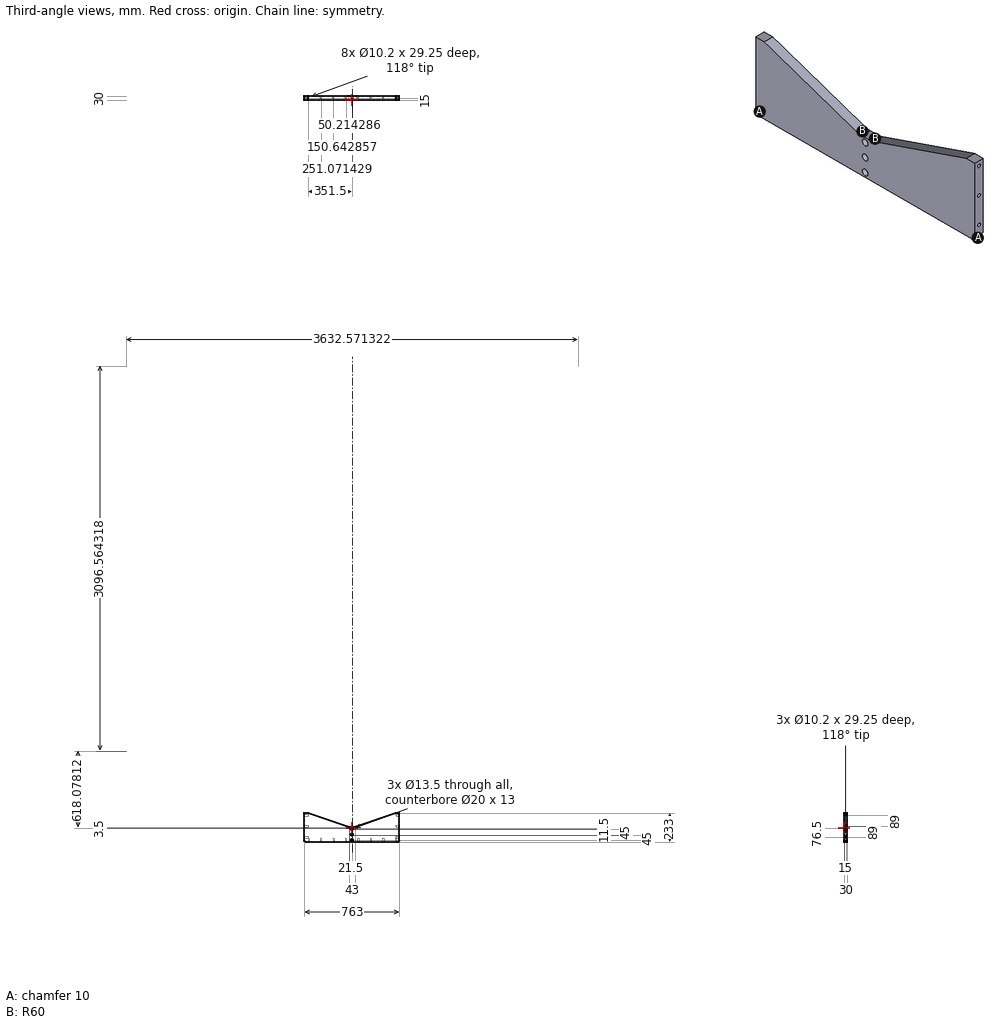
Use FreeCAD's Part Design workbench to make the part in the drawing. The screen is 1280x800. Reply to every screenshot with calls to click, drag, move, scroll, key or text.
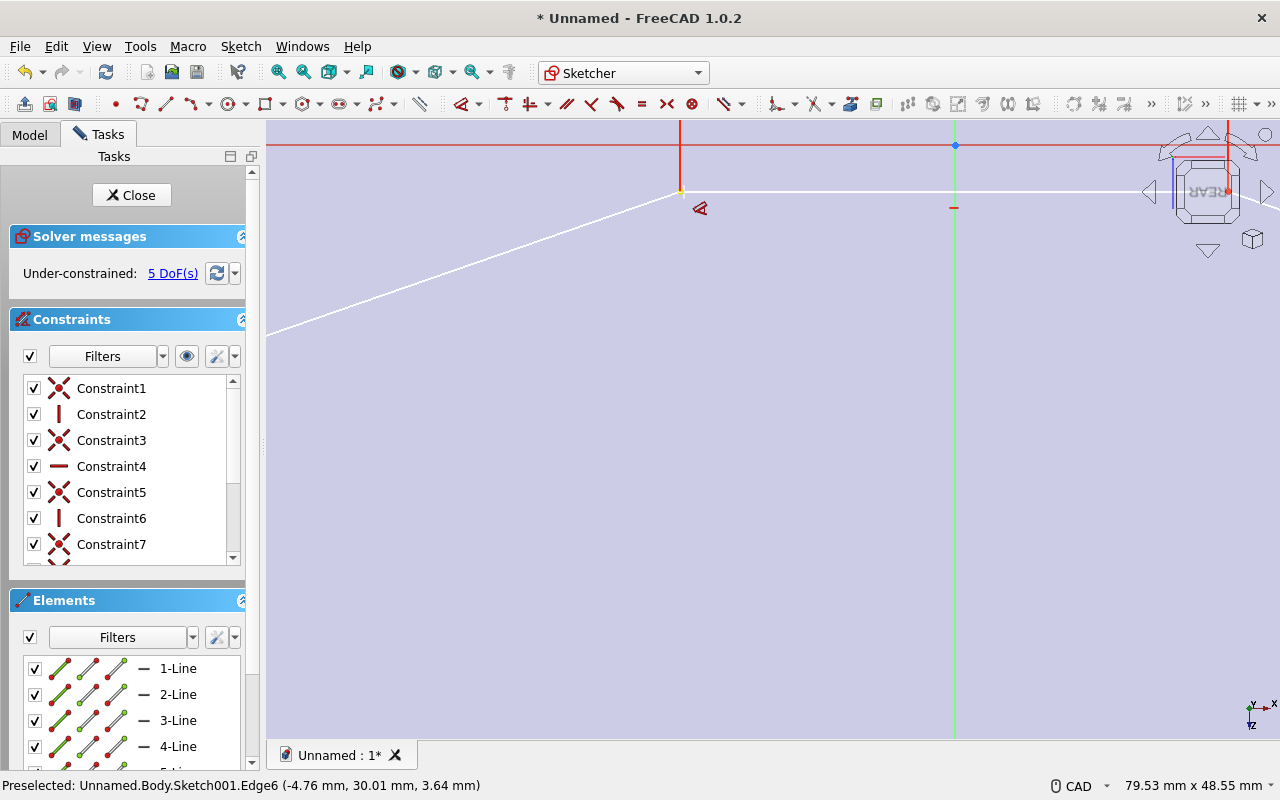
click(680, 192)
click(646, 170)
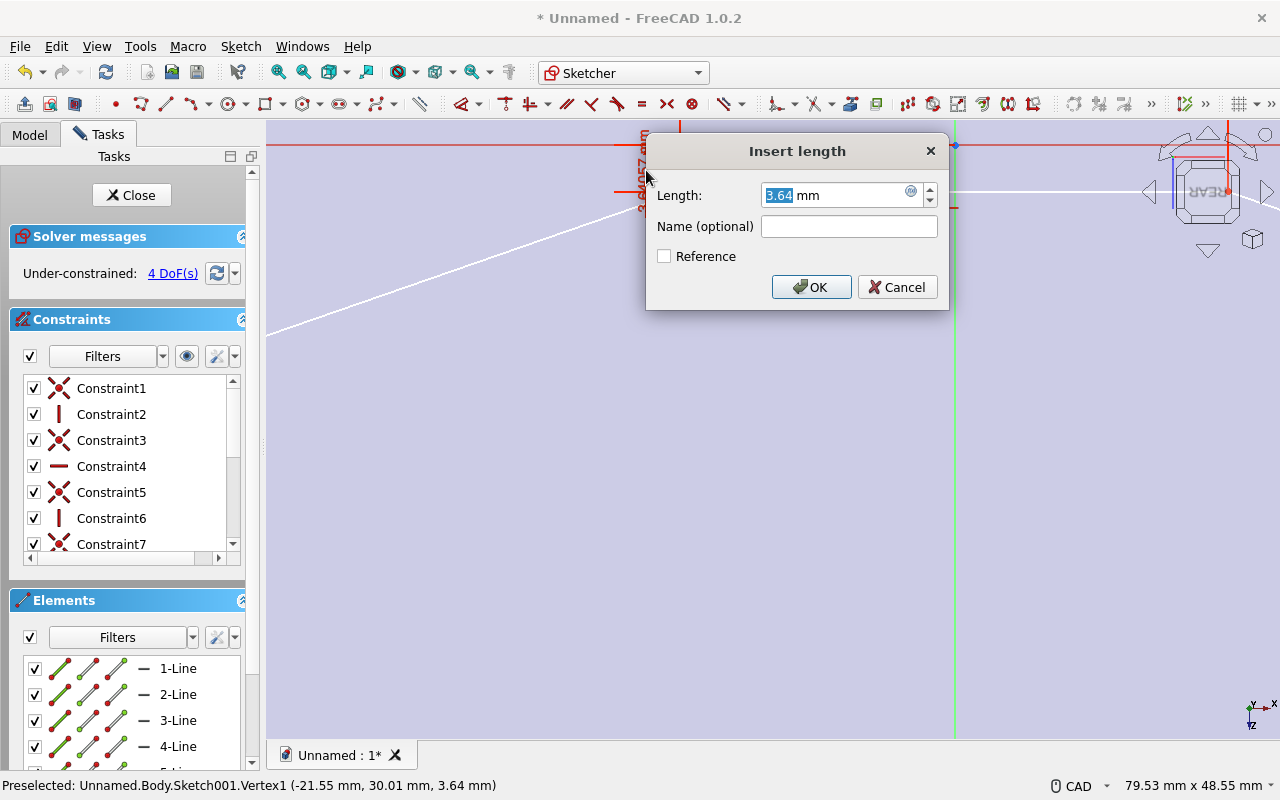
text(3.5)
key(Return)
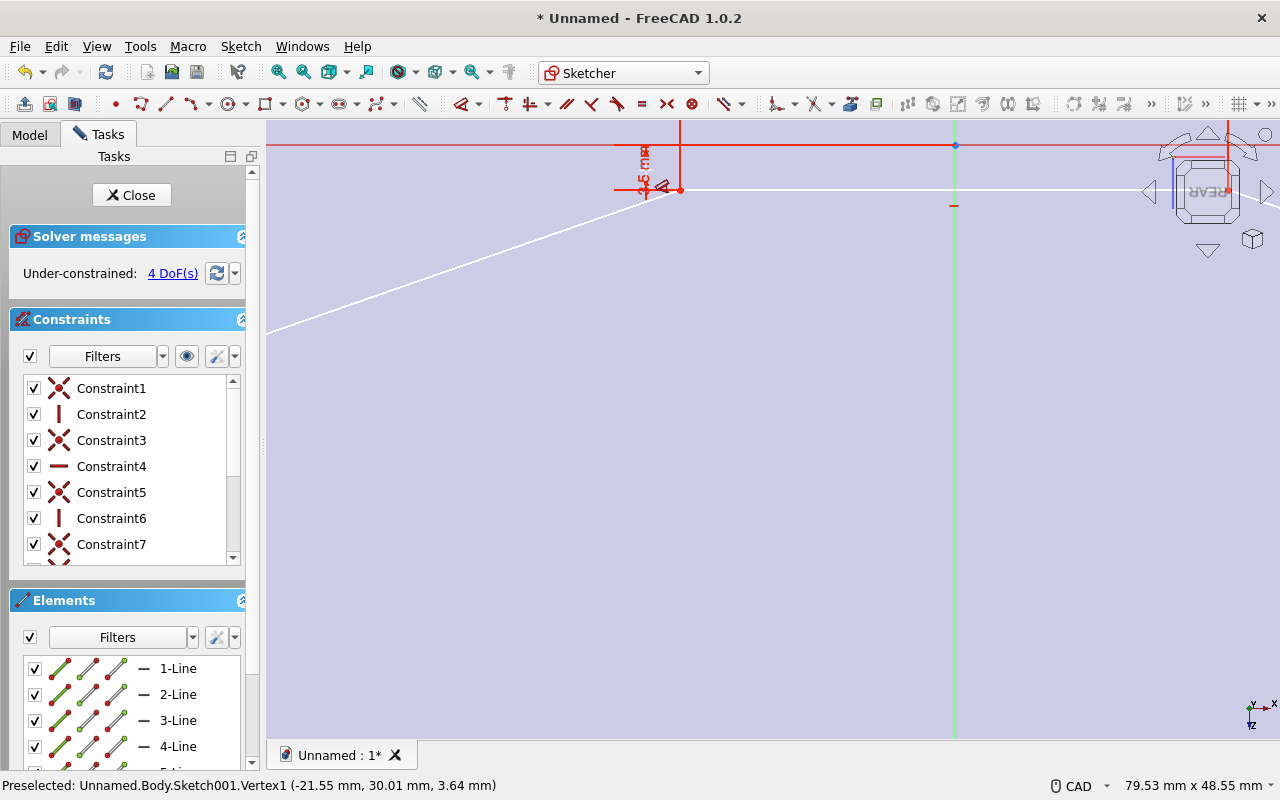
scroll(704, 430, down, 15)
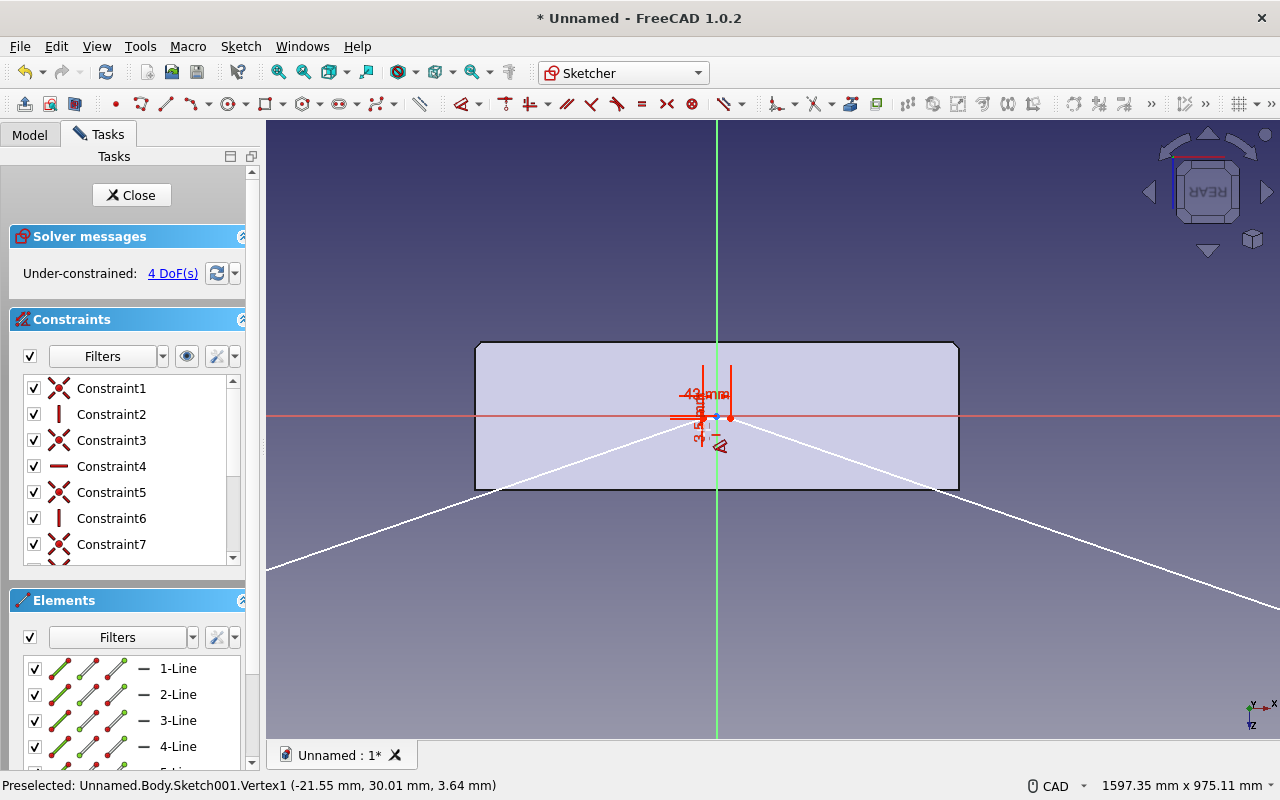
scroll(702, 199, down, 9)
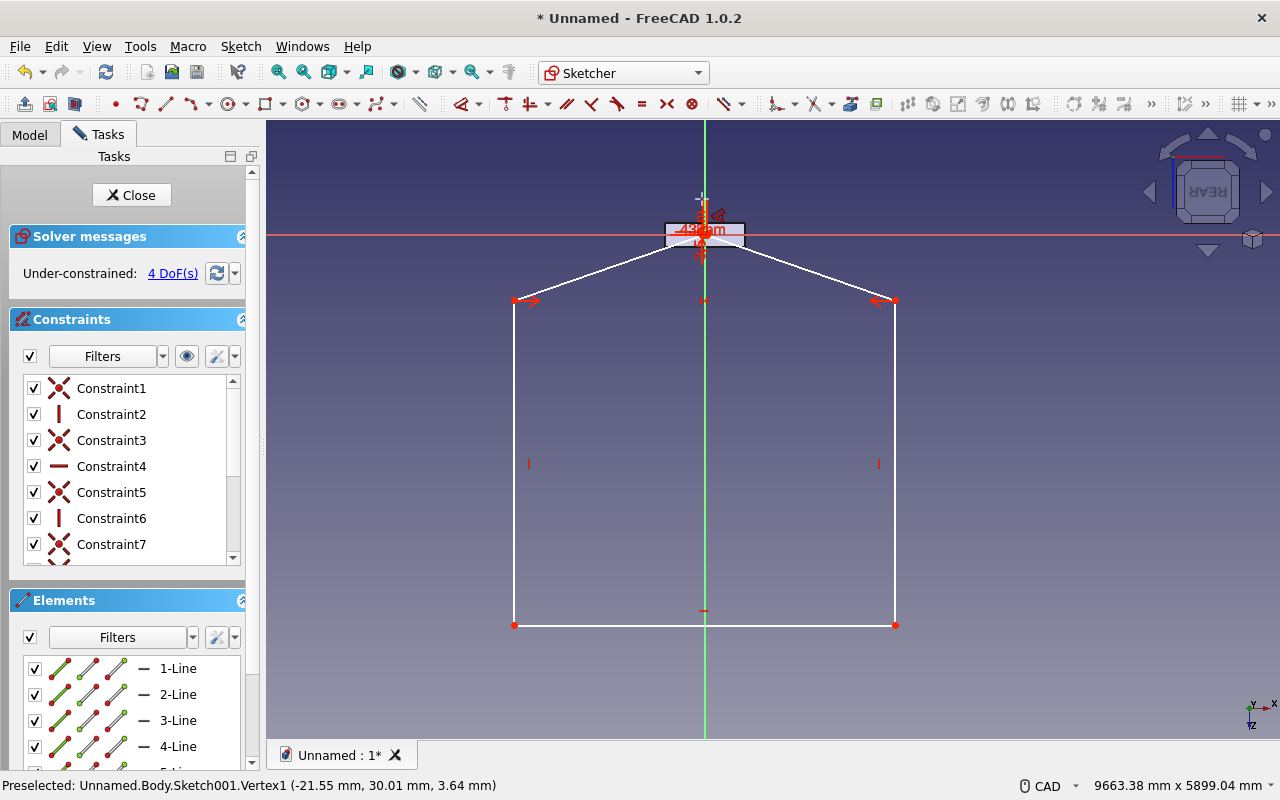
scroll(703, 235, up, 15)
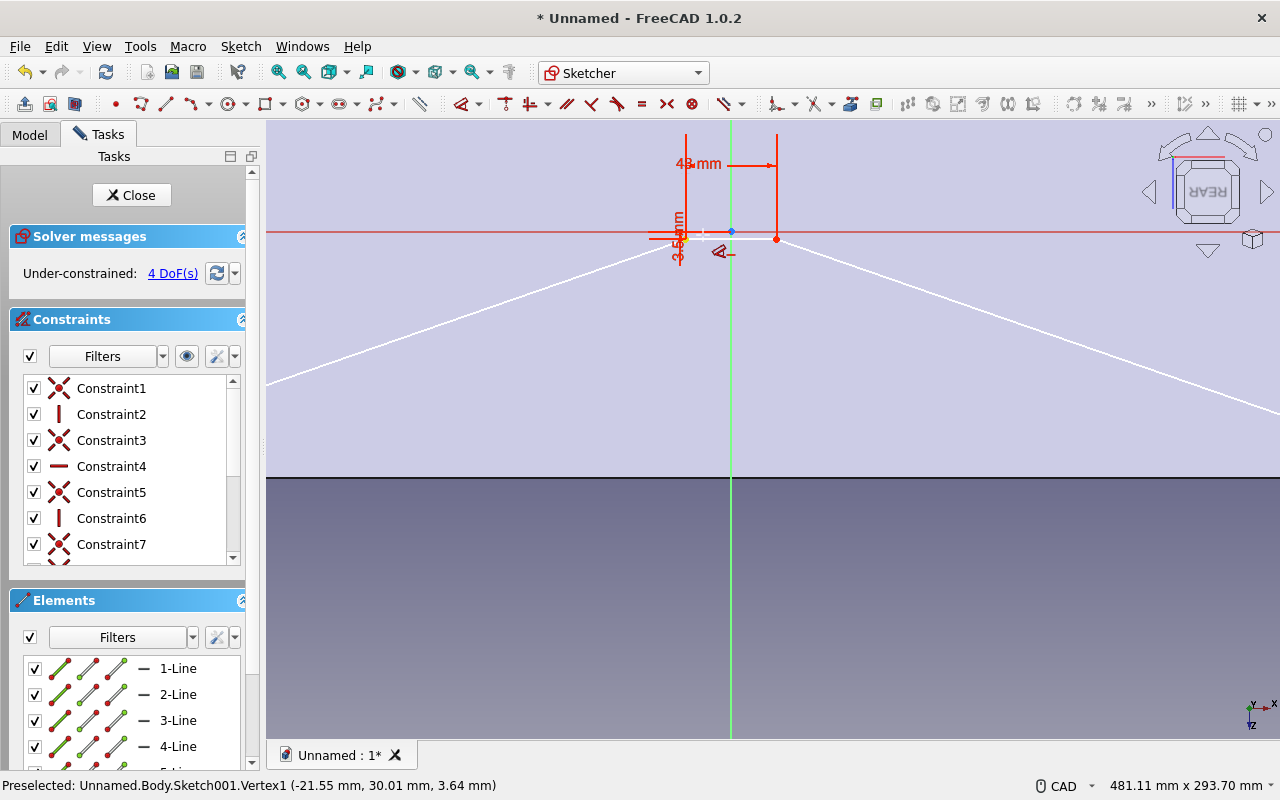
click(686, 239)
click(709, 198)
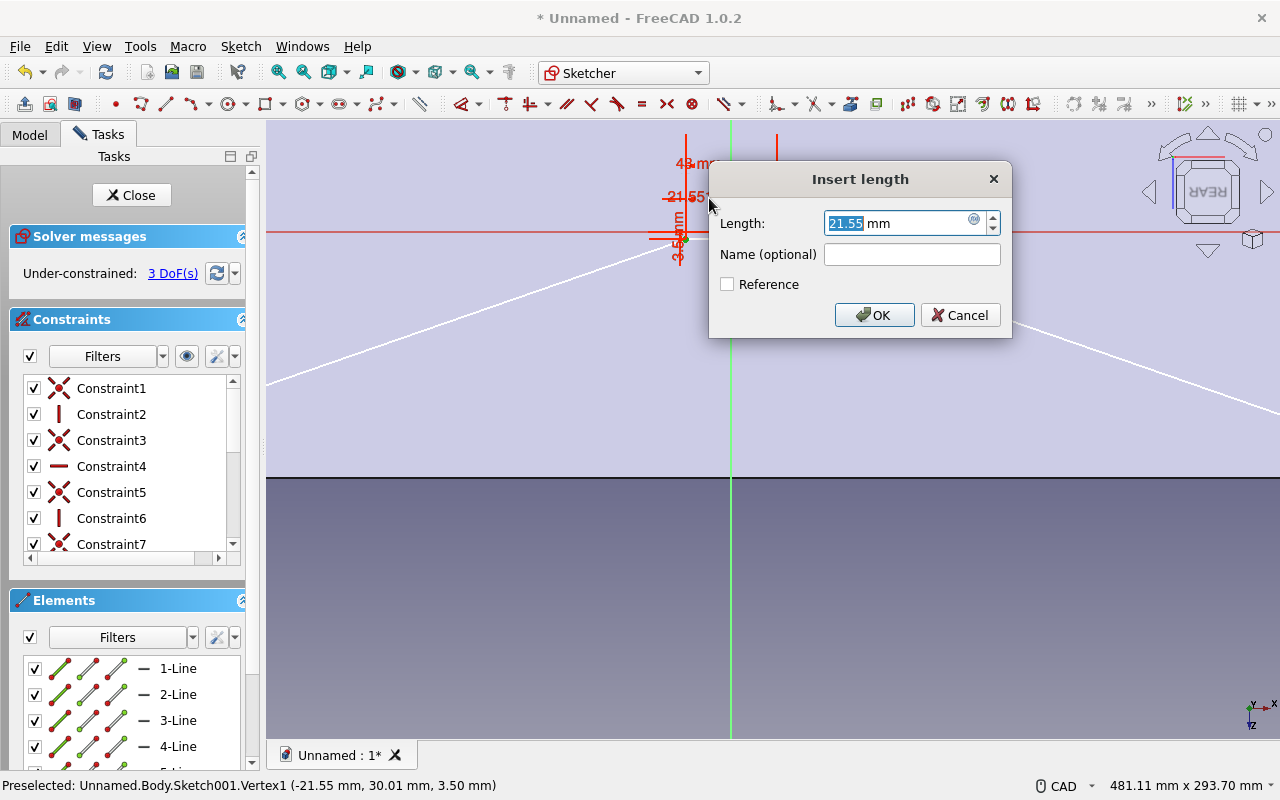
text(21.5)
key(Return)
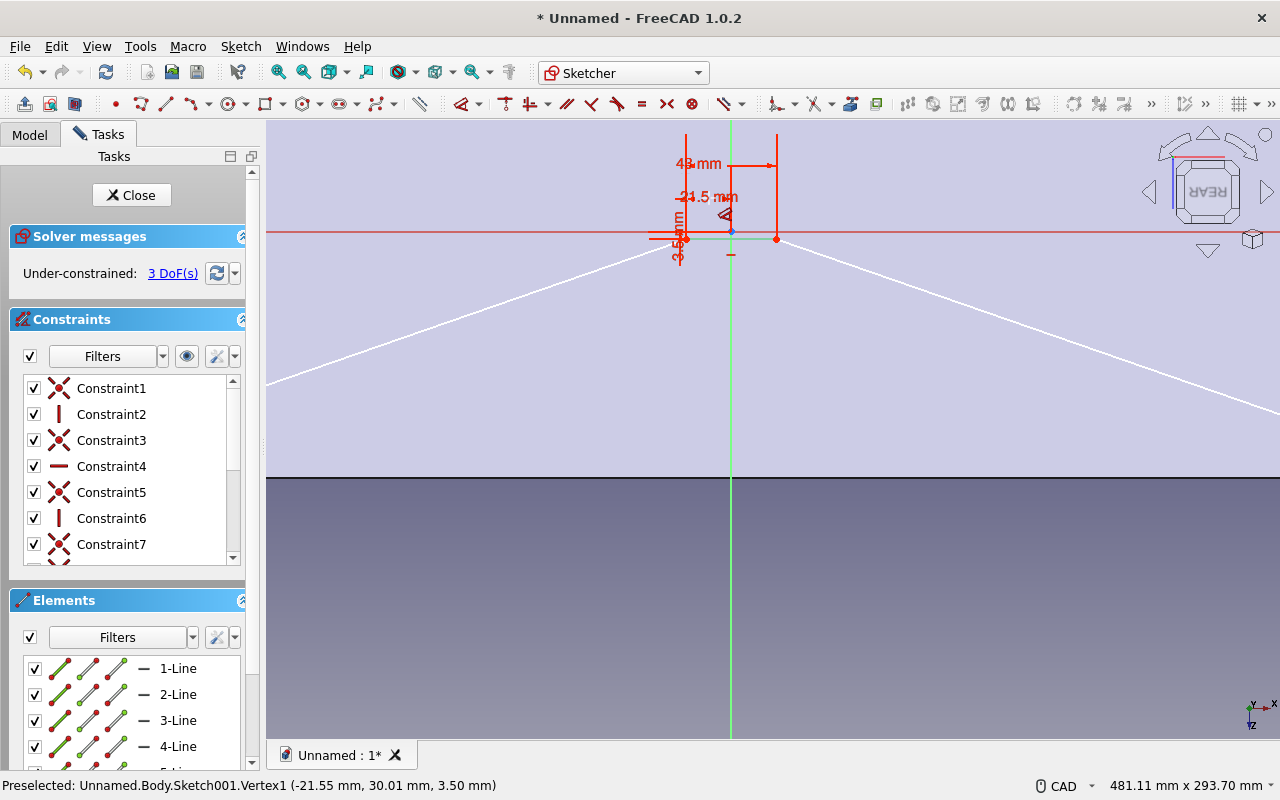
scroll(703, 235, down, 15)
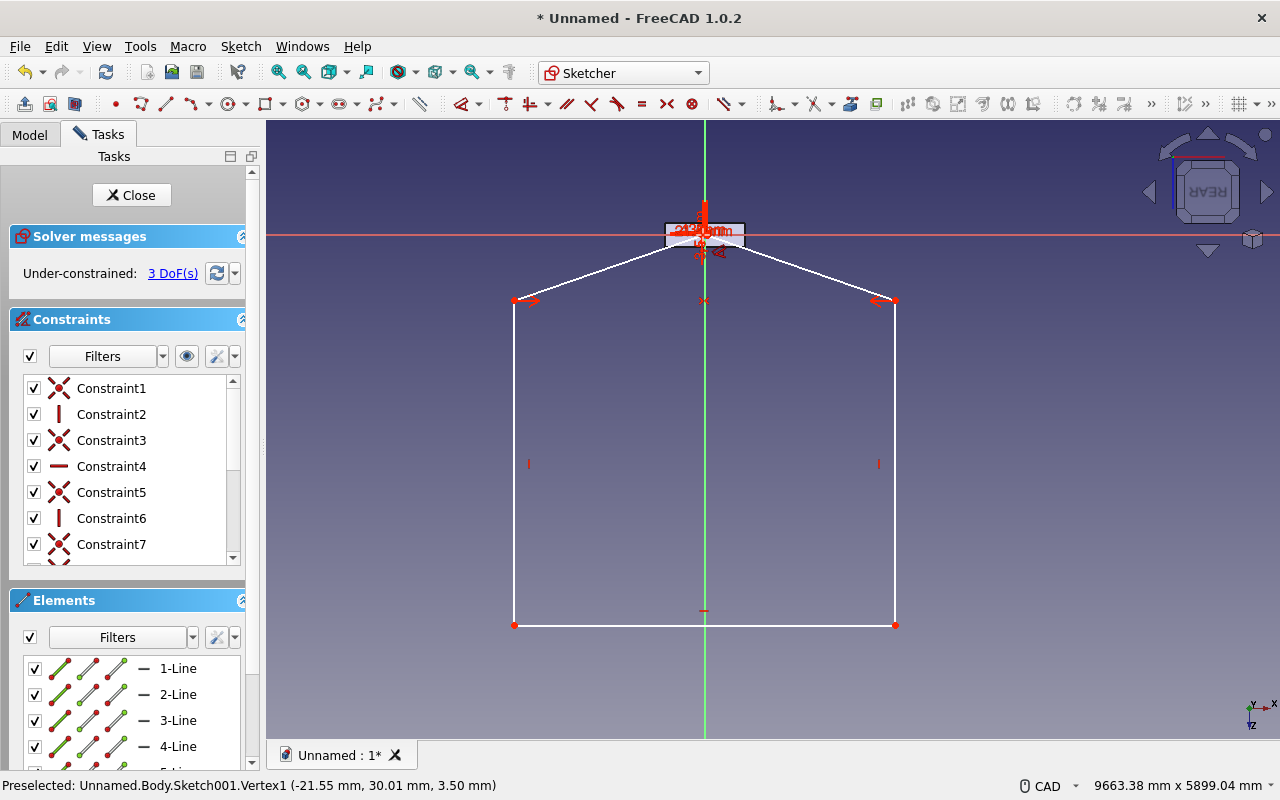
click(514, 301)
click(480, 268)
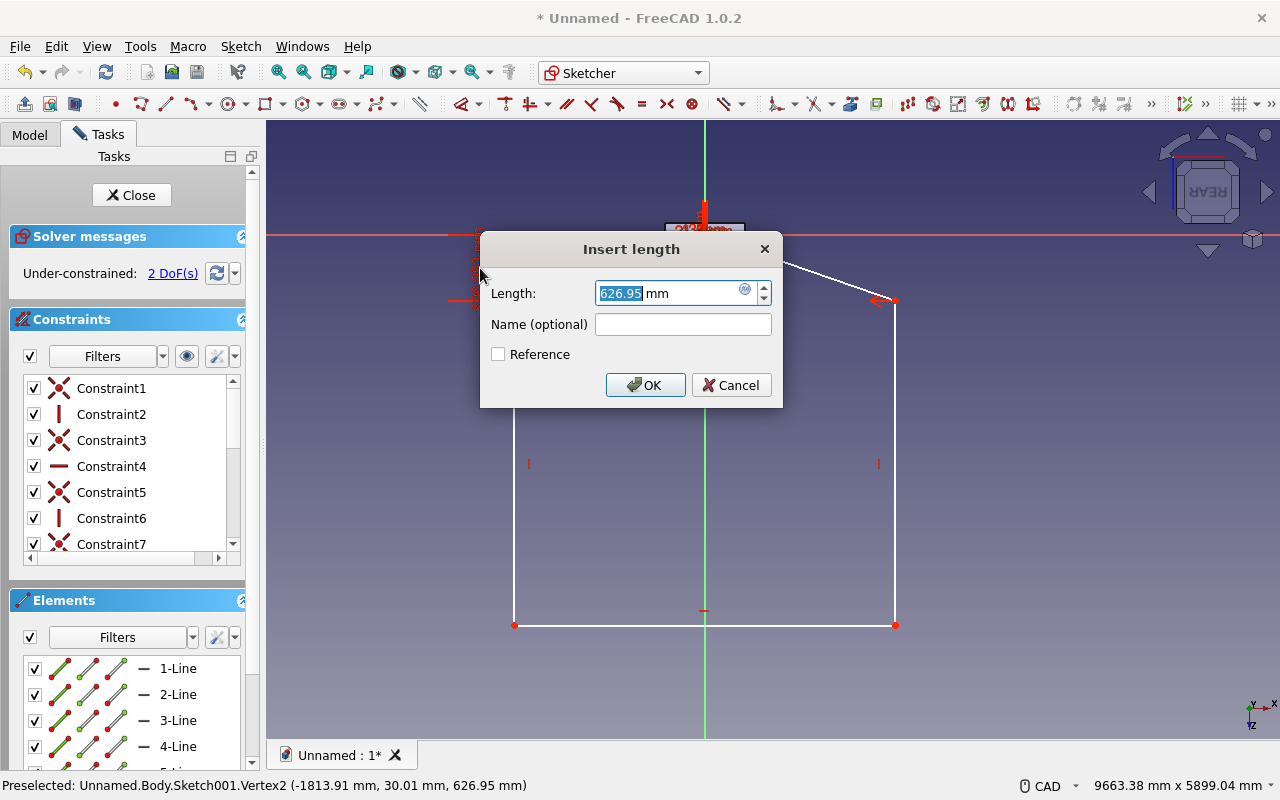
text(618.07812)
key(Return)